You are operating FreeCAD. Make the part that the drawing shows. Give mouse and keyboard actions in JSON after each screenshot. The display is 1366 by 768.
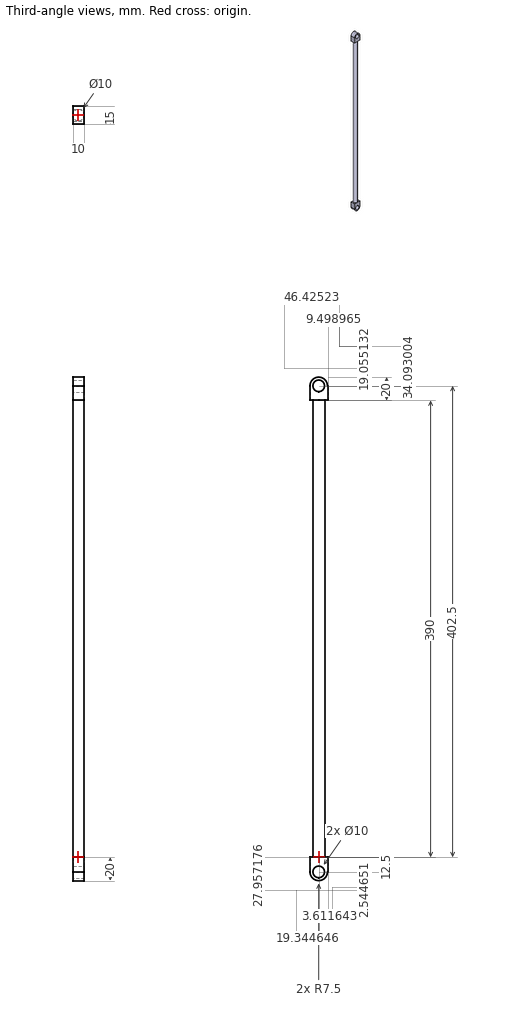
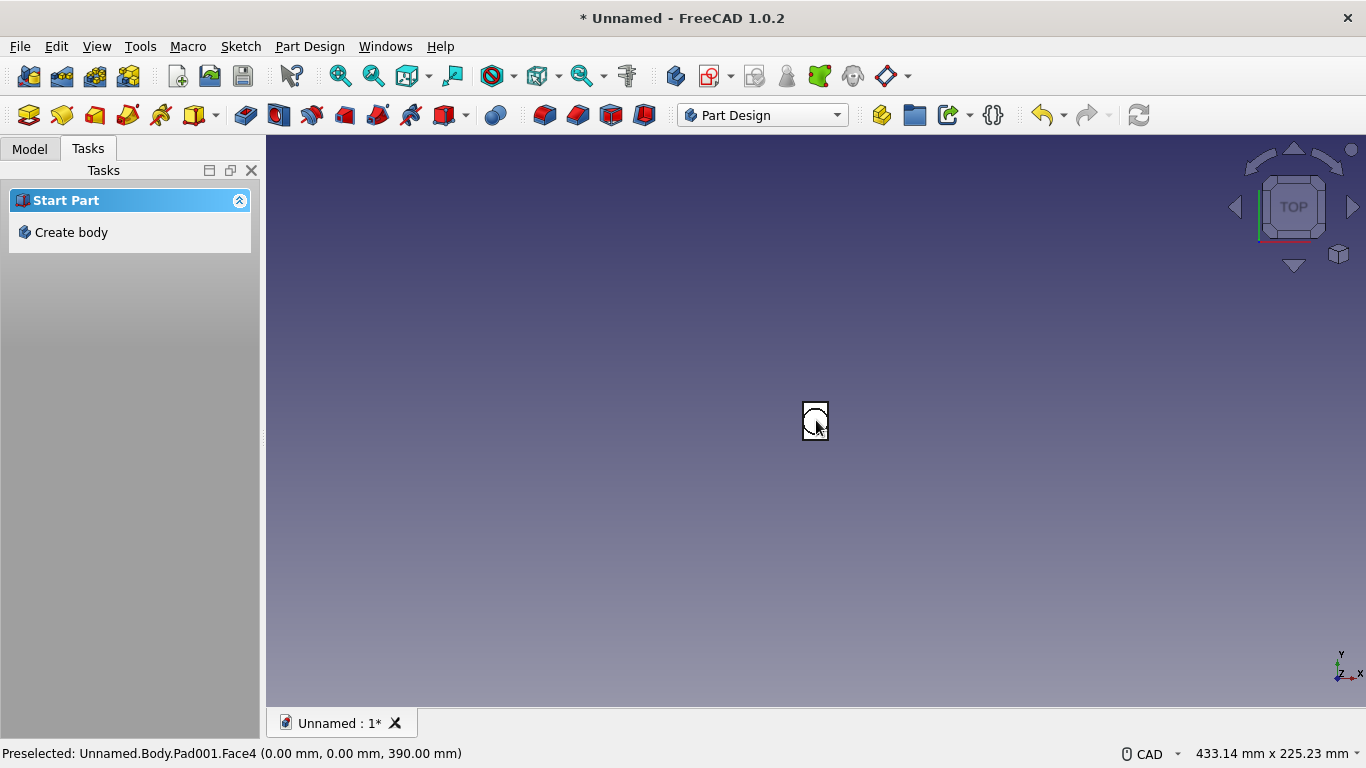
{"action": "left_click", "coordinate": [816, 420]}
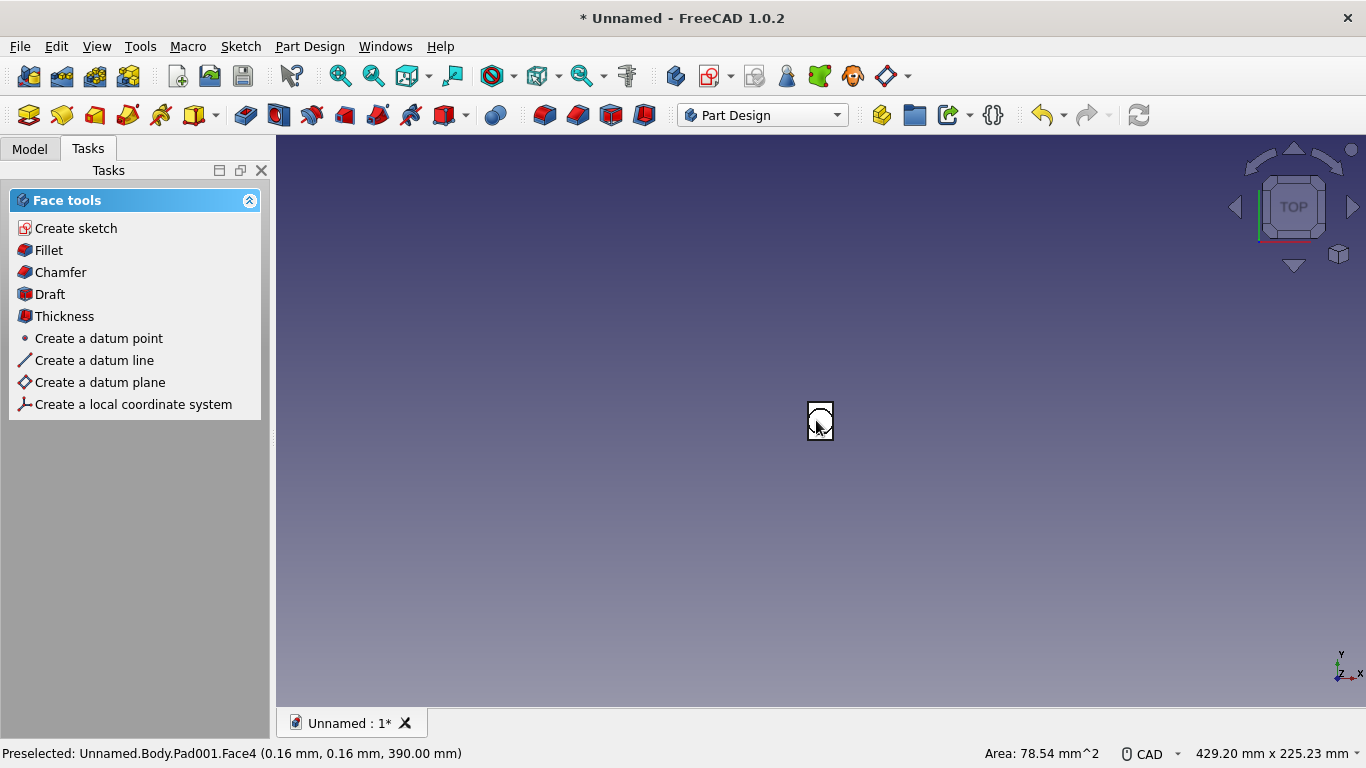
{"action": "left_click", "coordinate": [708, 76]}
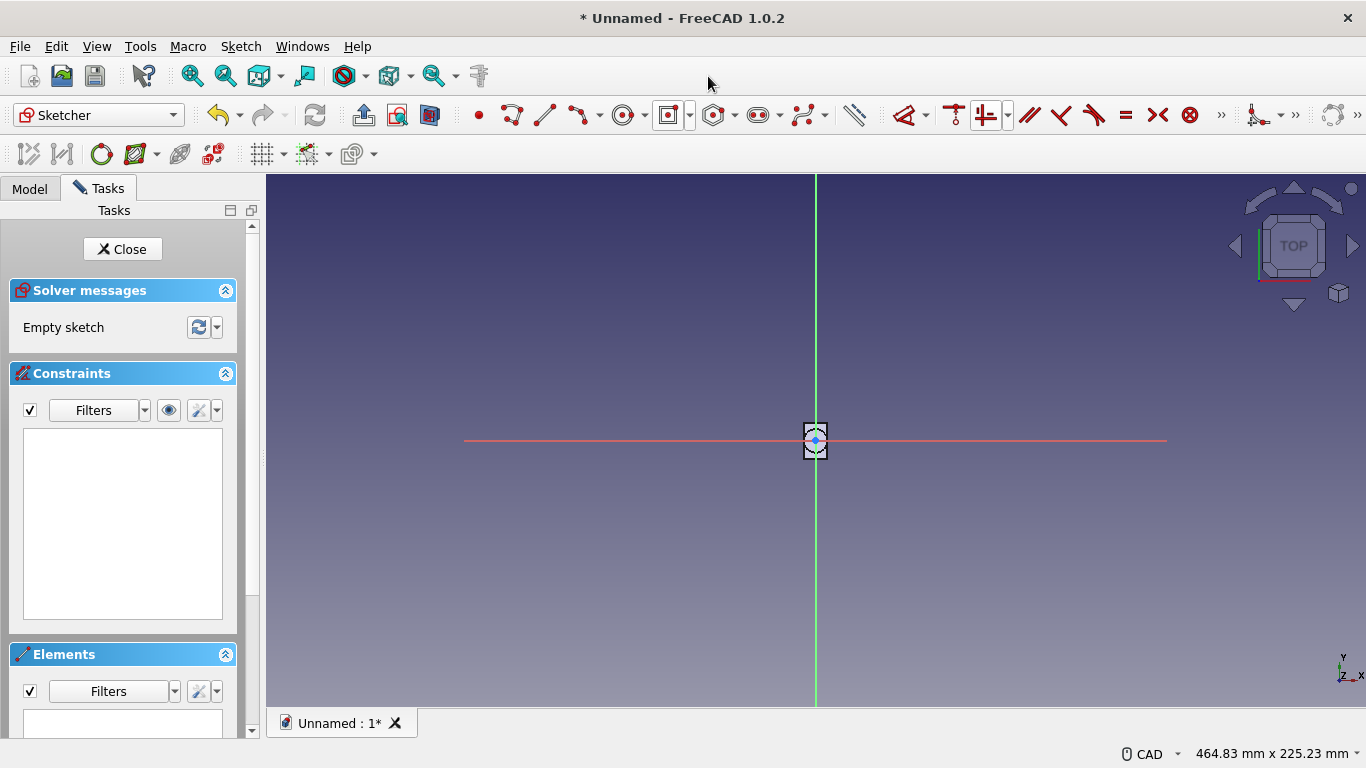
{"action": "scroll", "coordinate": [824, 441], "scroll_direction": "up", "scroll_amount": 11}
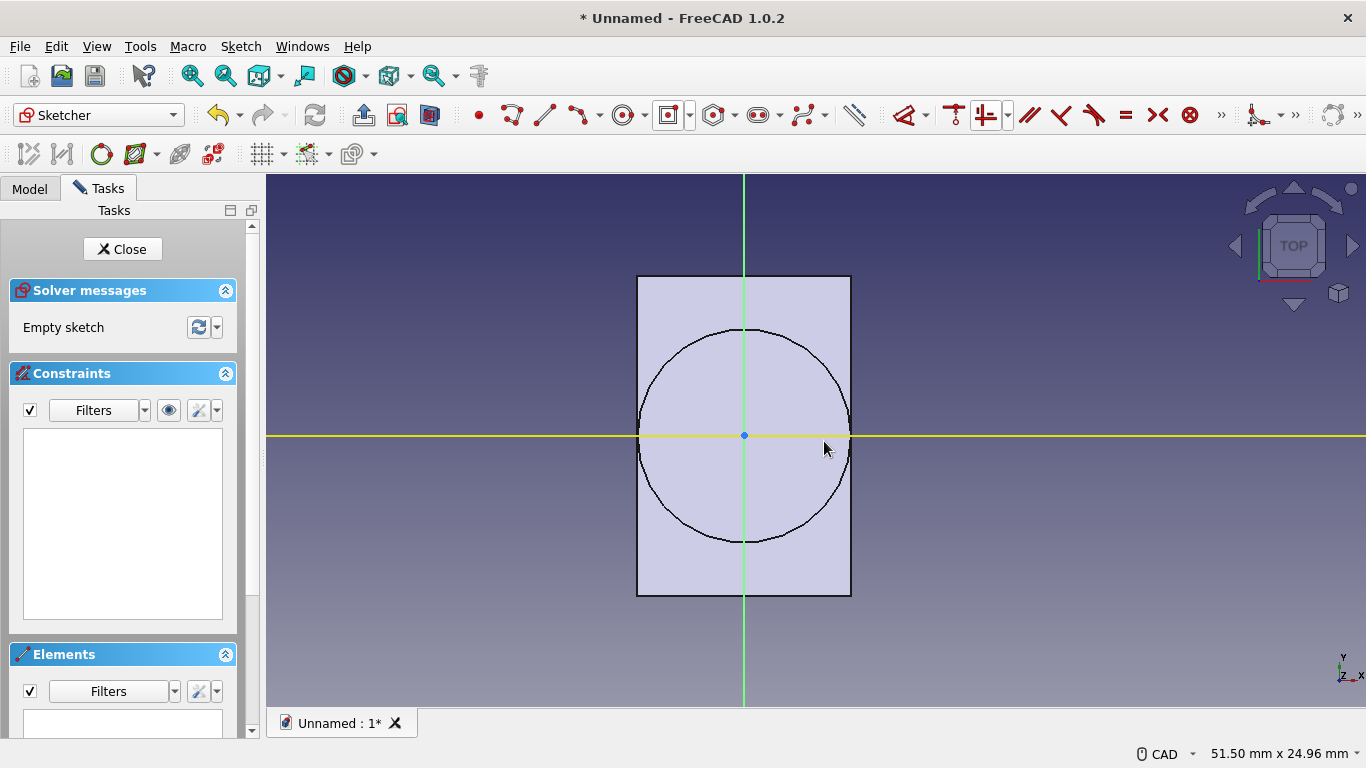
{"action": "left_click", "coordinate": [668, 116]}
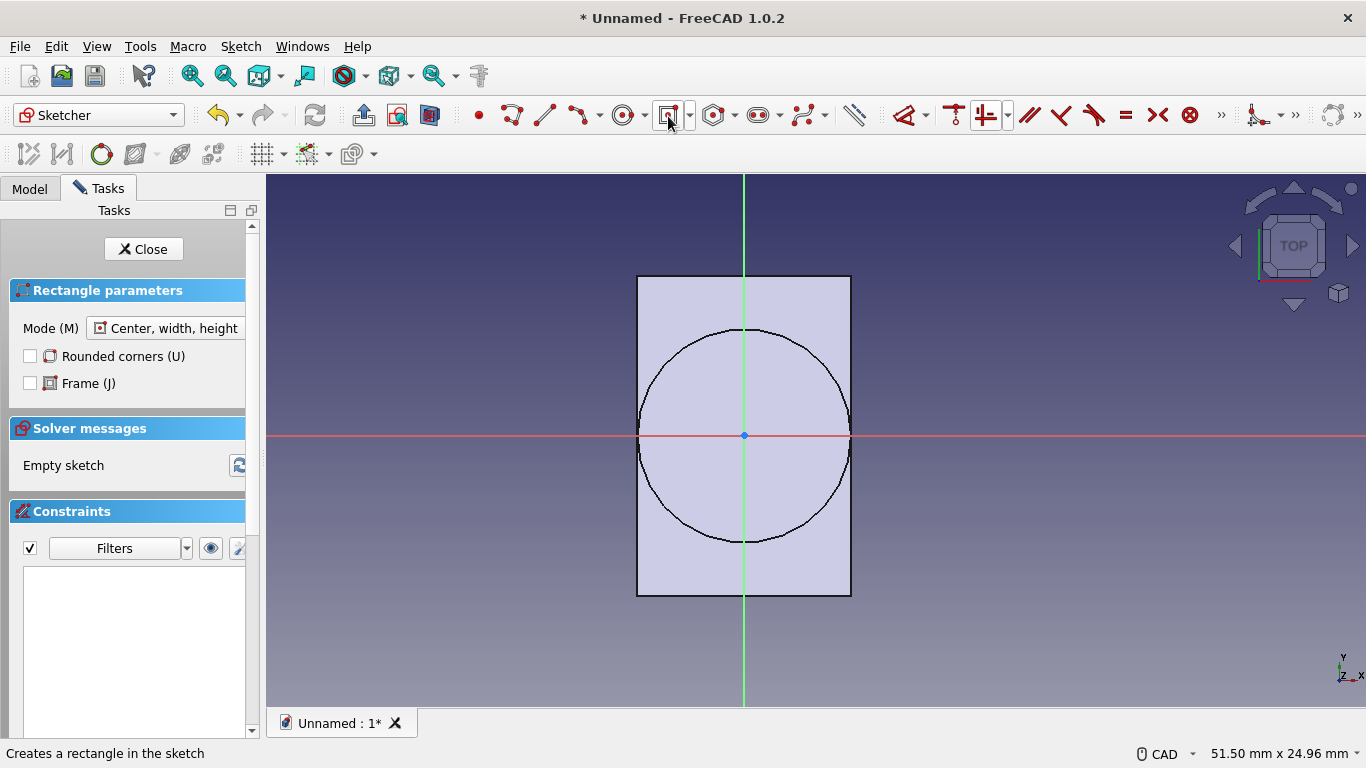
{"action": "left_click", "coordinate": [744, 436]}
{"action": "mouse_move", "coordinate": [851, 276]}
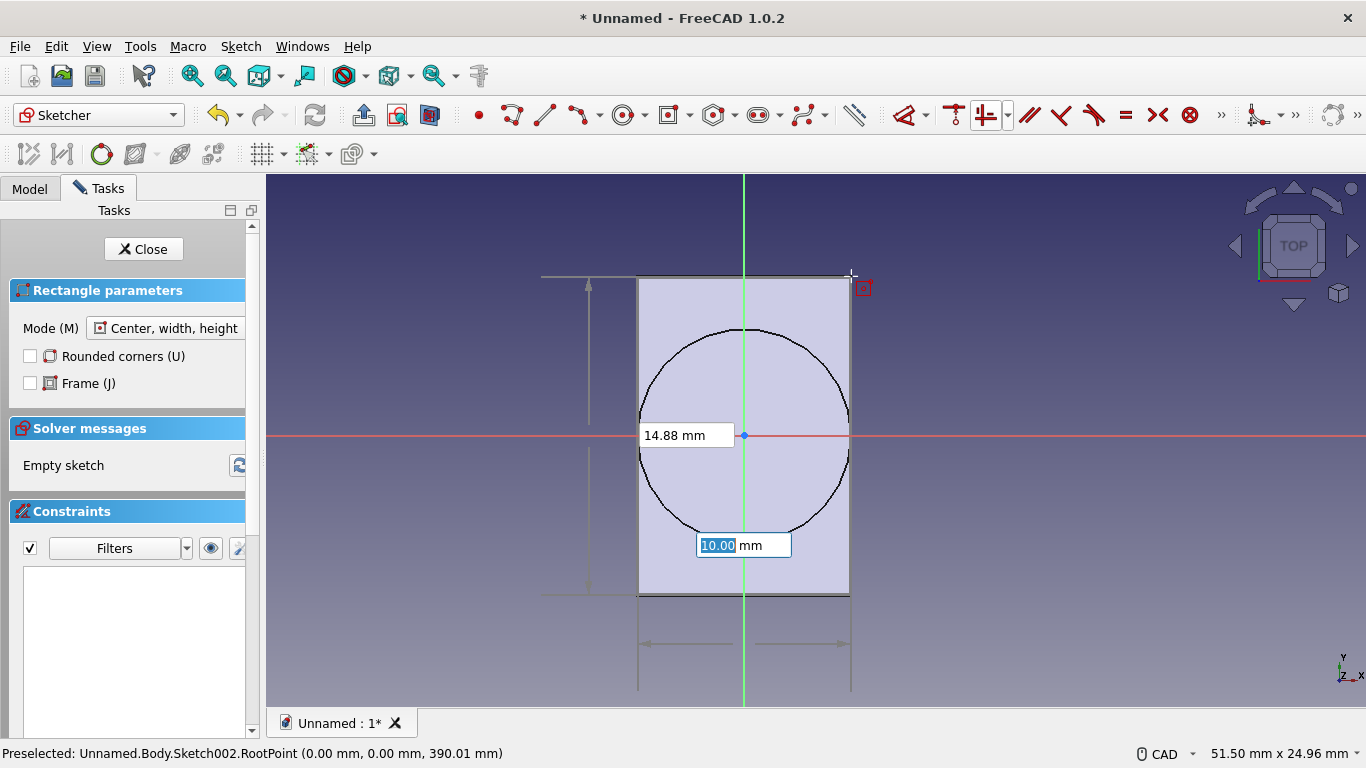
{"action": "type", "text": "10"}
{"action": "key", "text": "Tab"}
{"action": "type", "text": "15"}
{"action": "key", "text": "Return"}
{"action": "key", "text": "Escape"}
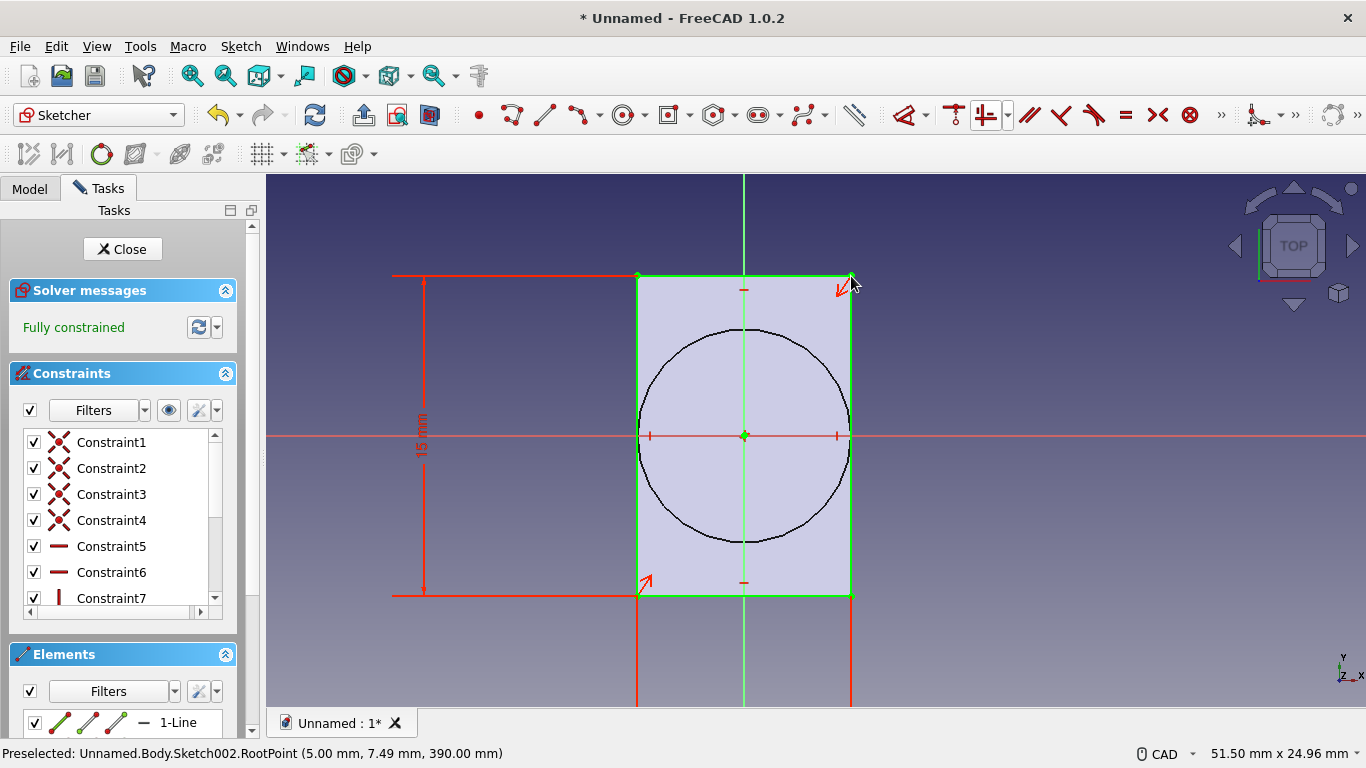
{"action": "left_click", "coordinate": [123, 249]}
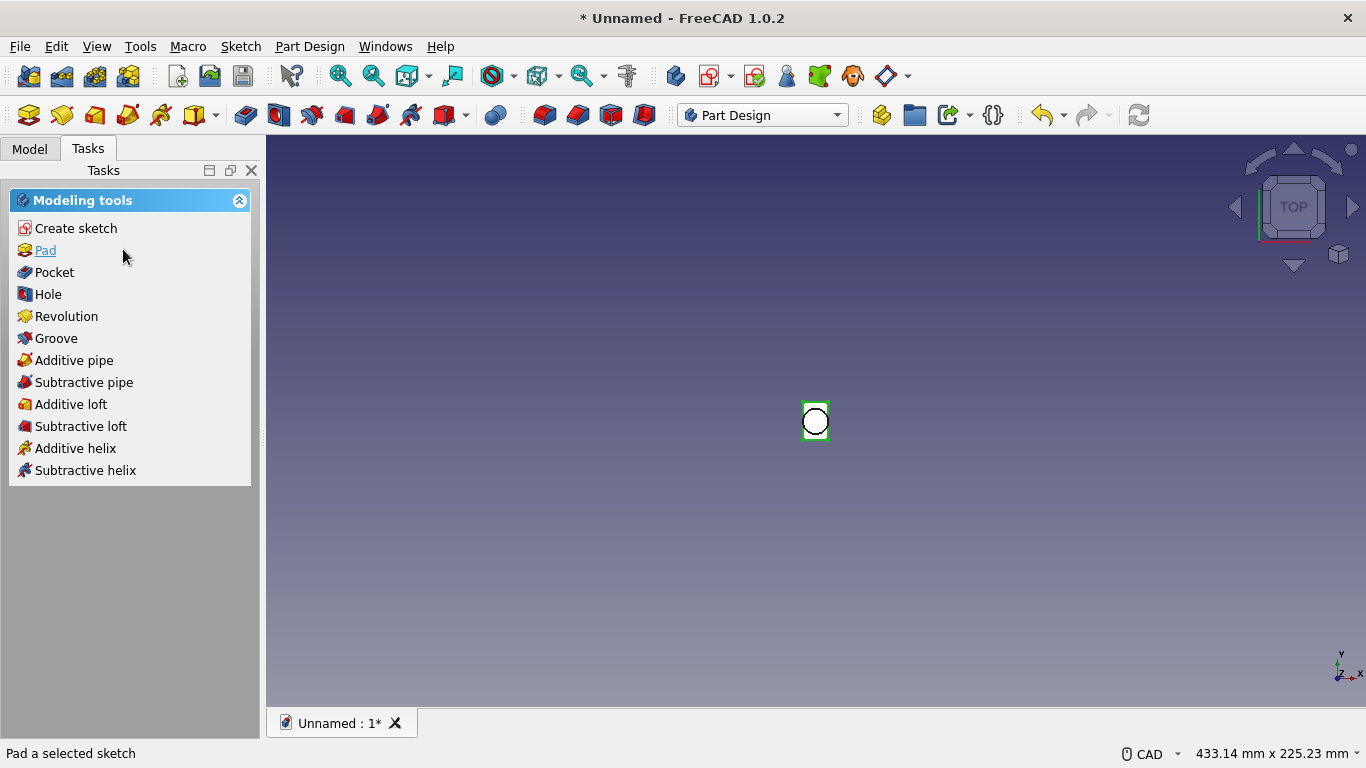
{"action": "left_click", "coordinate": [29, 116]}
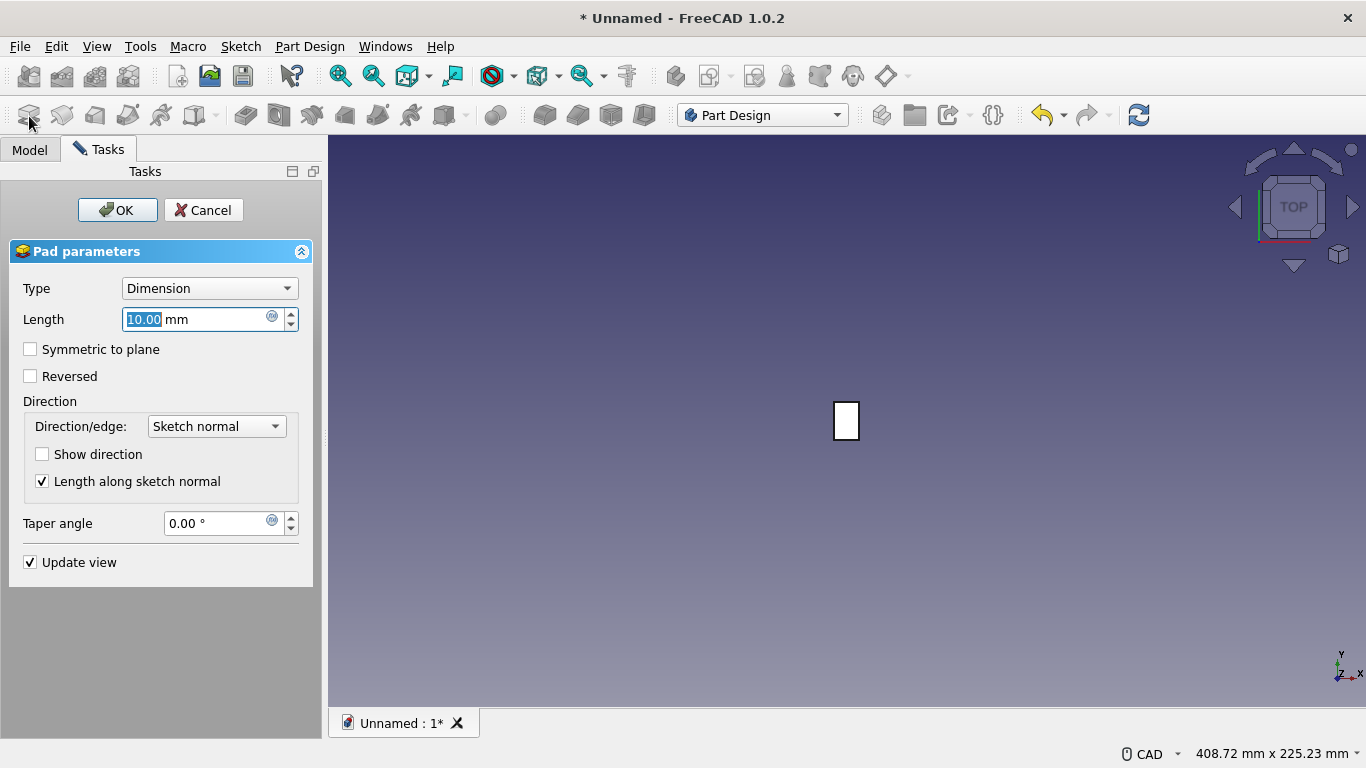
{"action": "type", "text": "20"}
{"action": "key", "text": "Tab"}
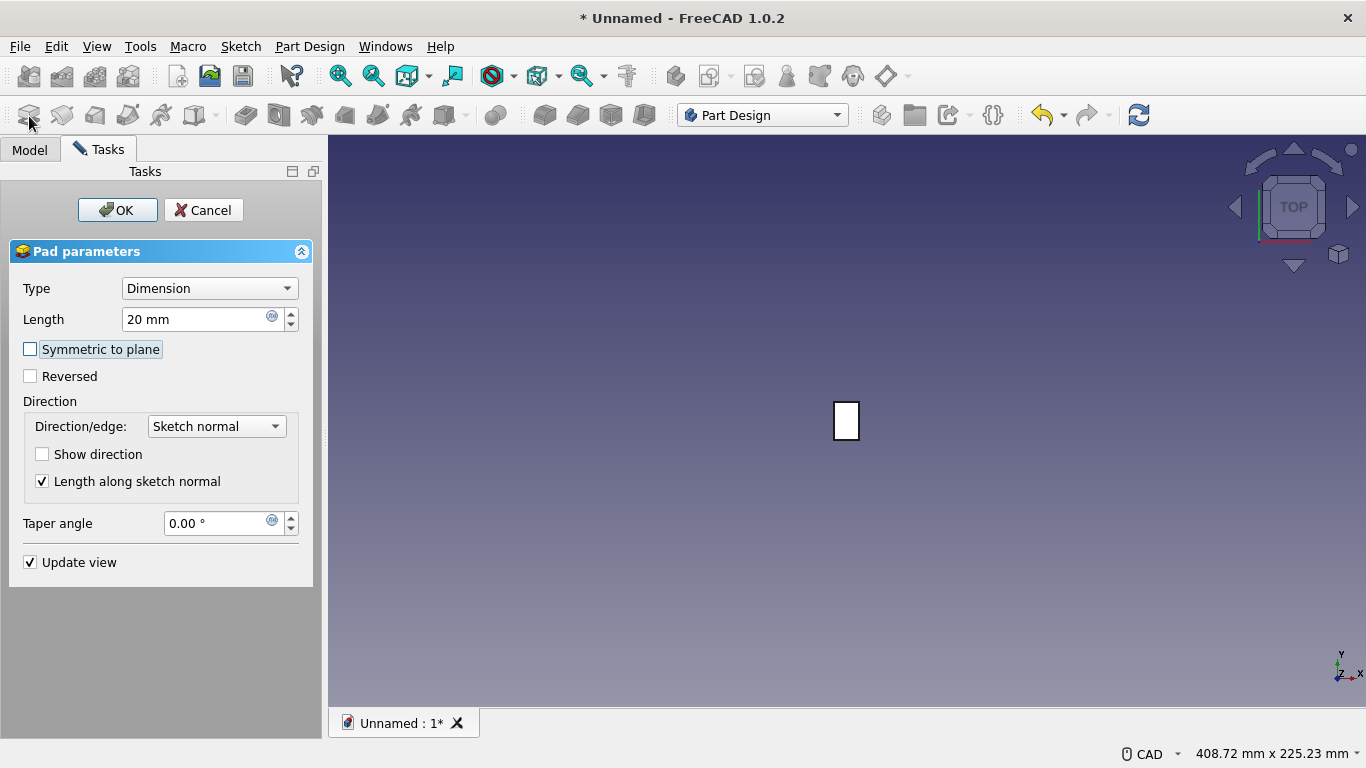
{"action": "left_click", "coordinate": [118, 210]}